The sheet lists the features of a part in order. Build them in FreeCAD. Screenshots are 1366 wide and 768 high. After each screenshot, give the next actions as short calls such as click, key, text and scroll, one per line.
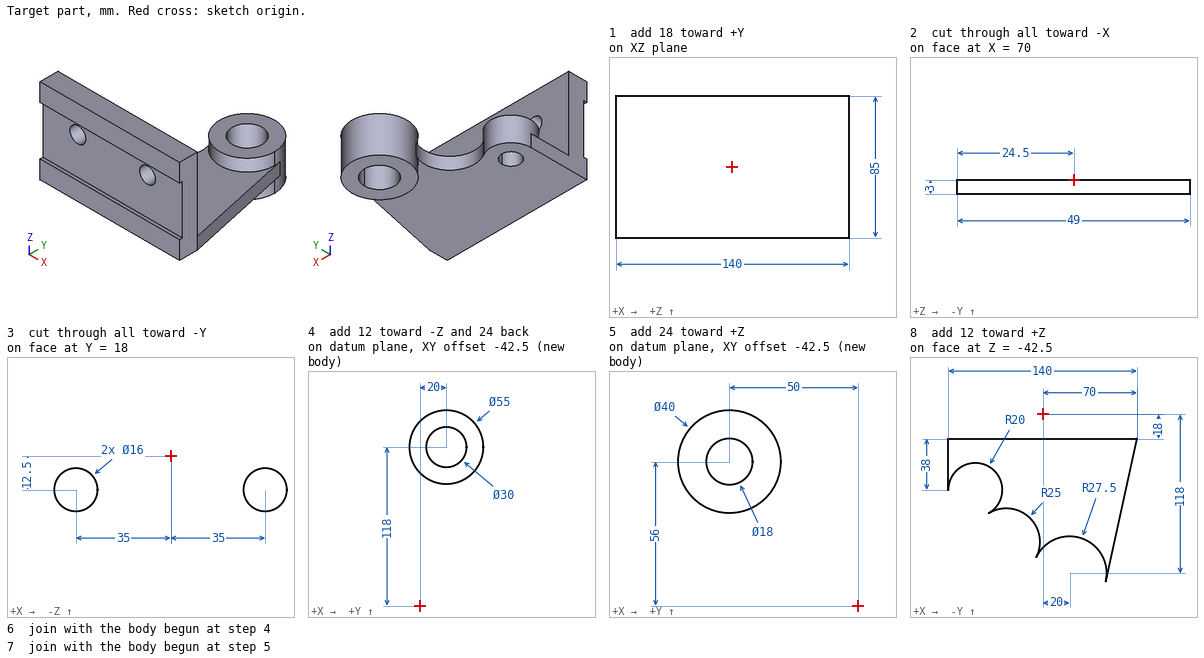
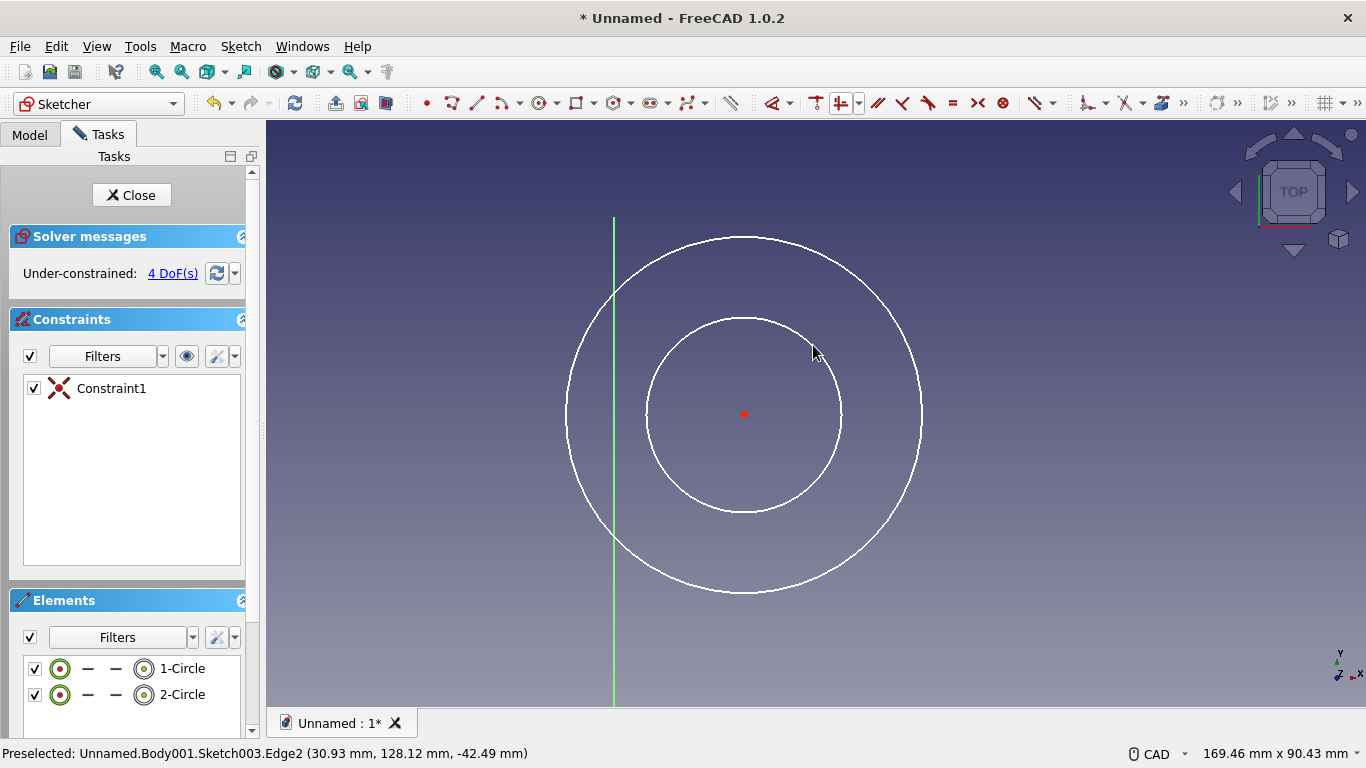
click(772, 104)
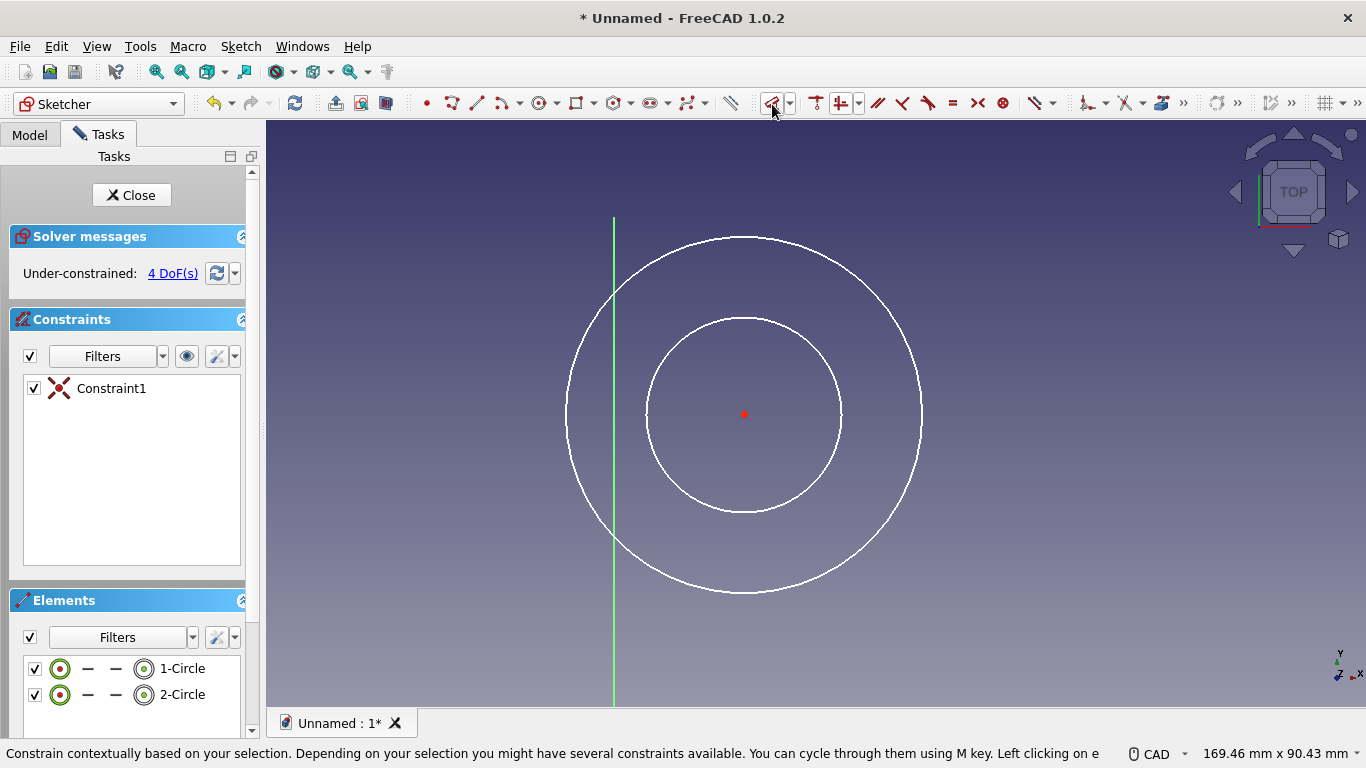
click(870, 289)
click(893, 266)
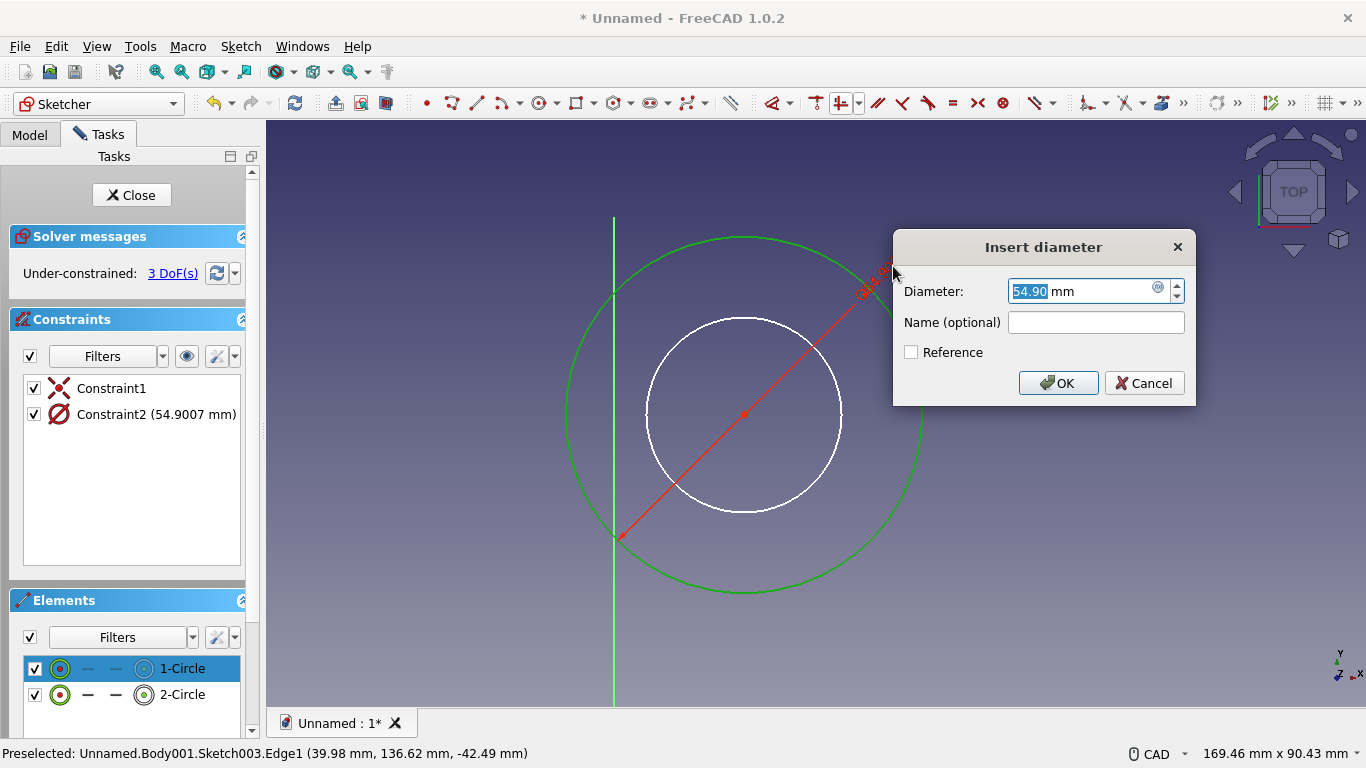
text(55)
key(Return)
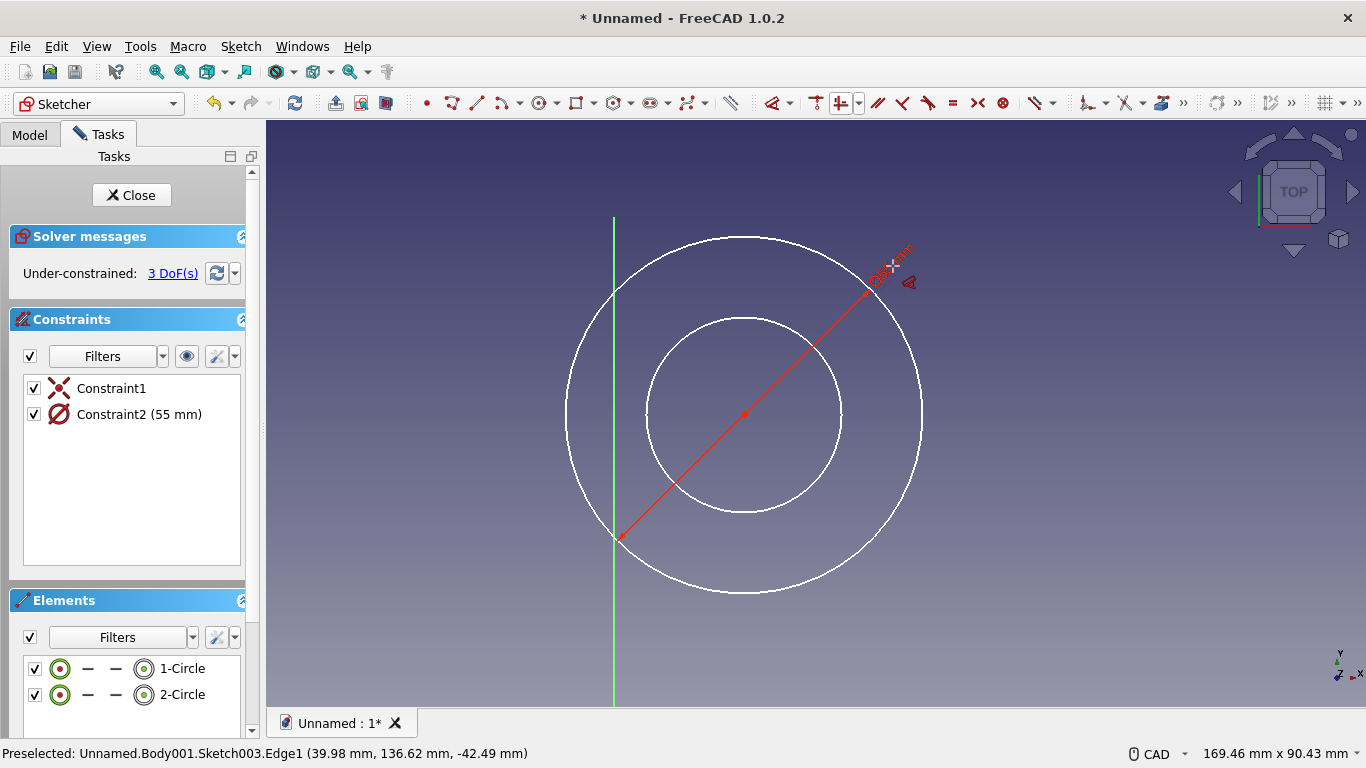
click(813, 346)
click(836, 323)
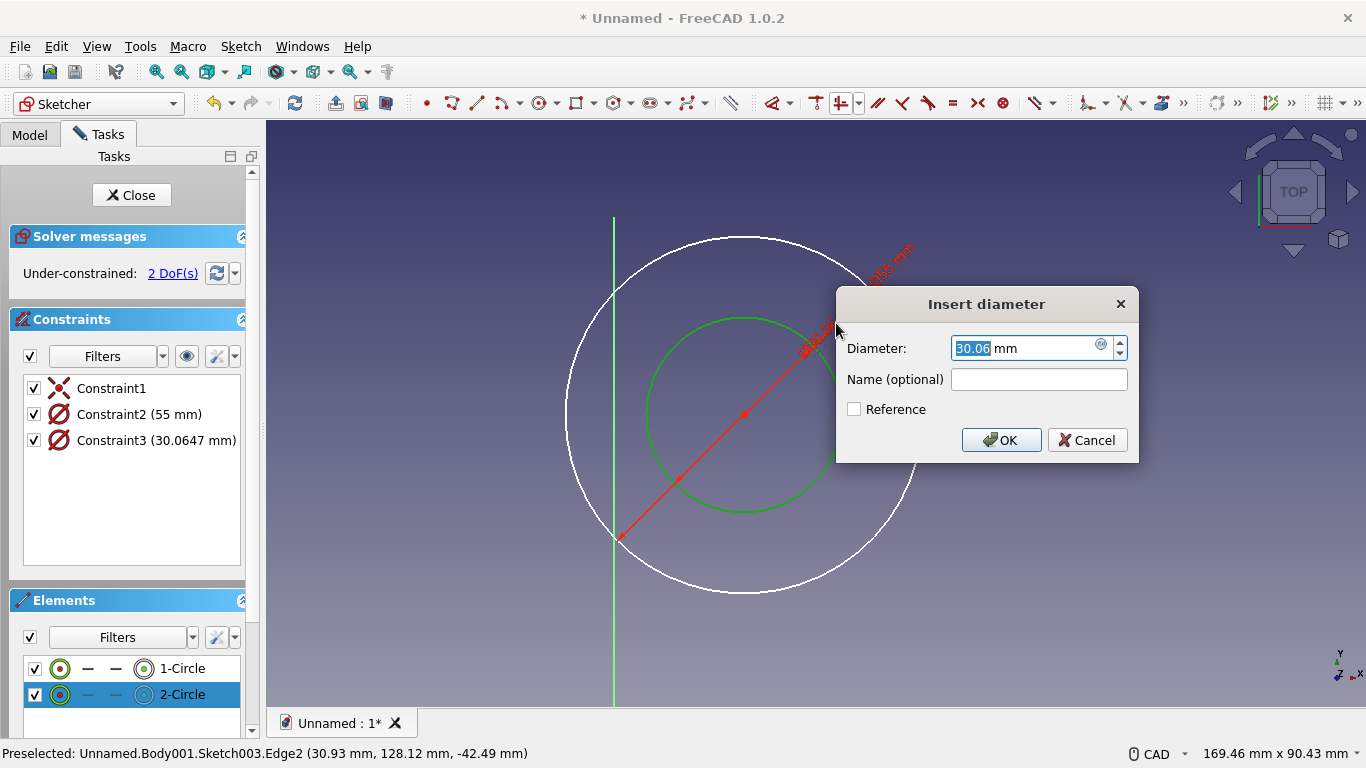
text(30)
key(Return)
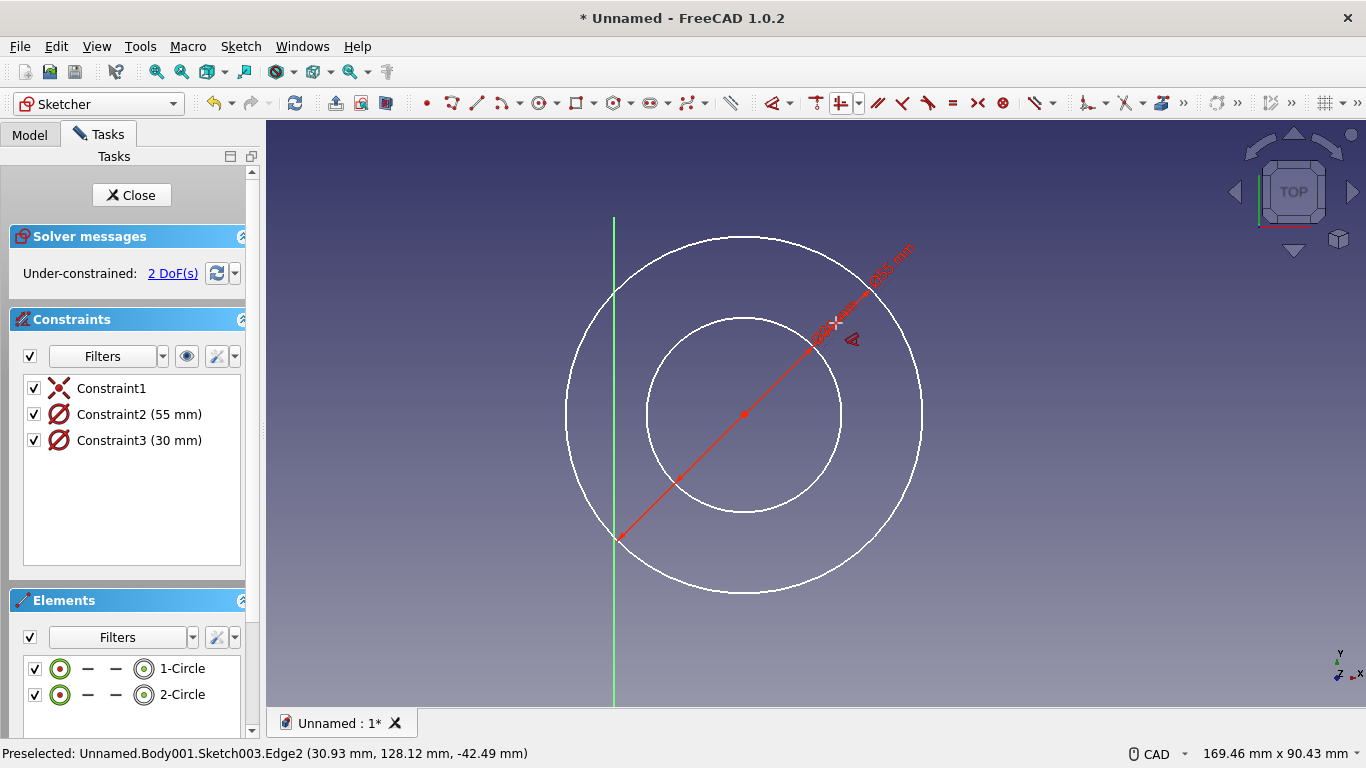
click(744, 415)
click(679, 381)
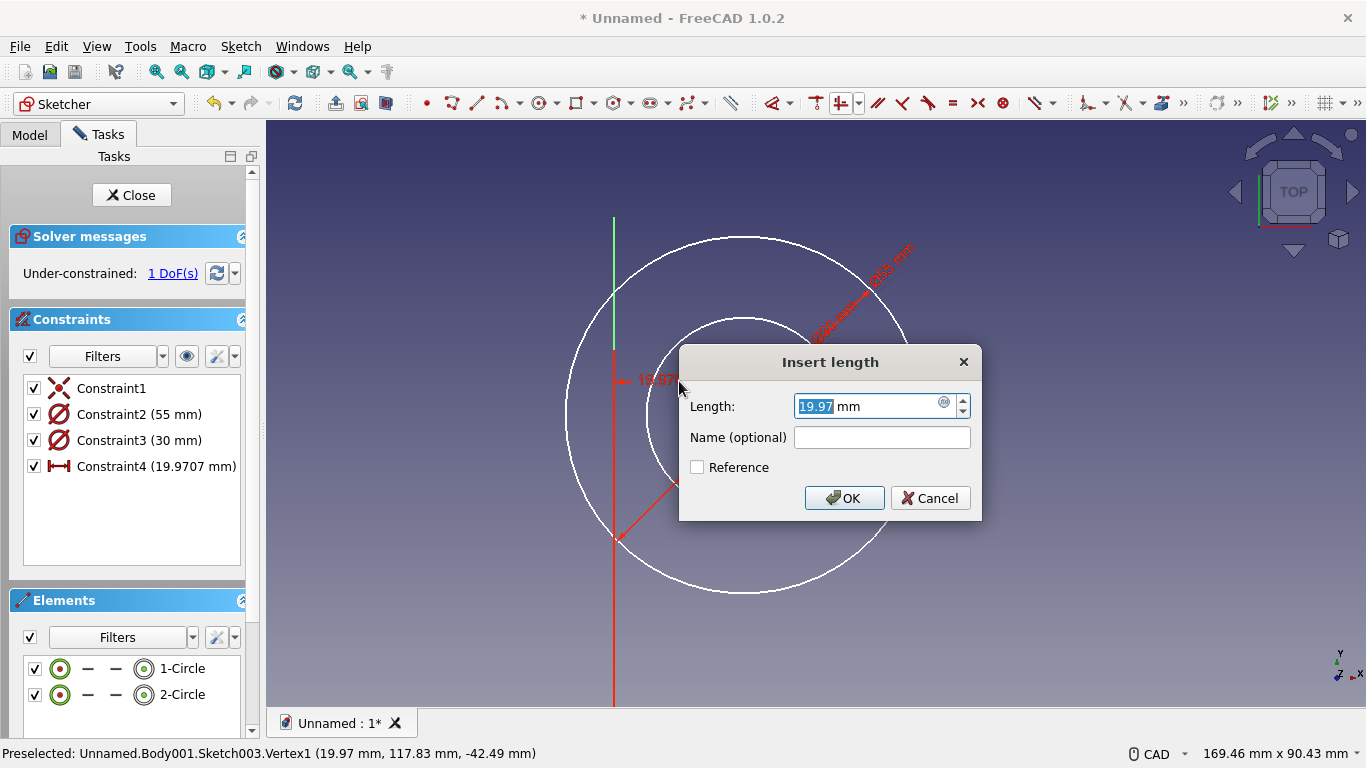
text(20)
key(Return)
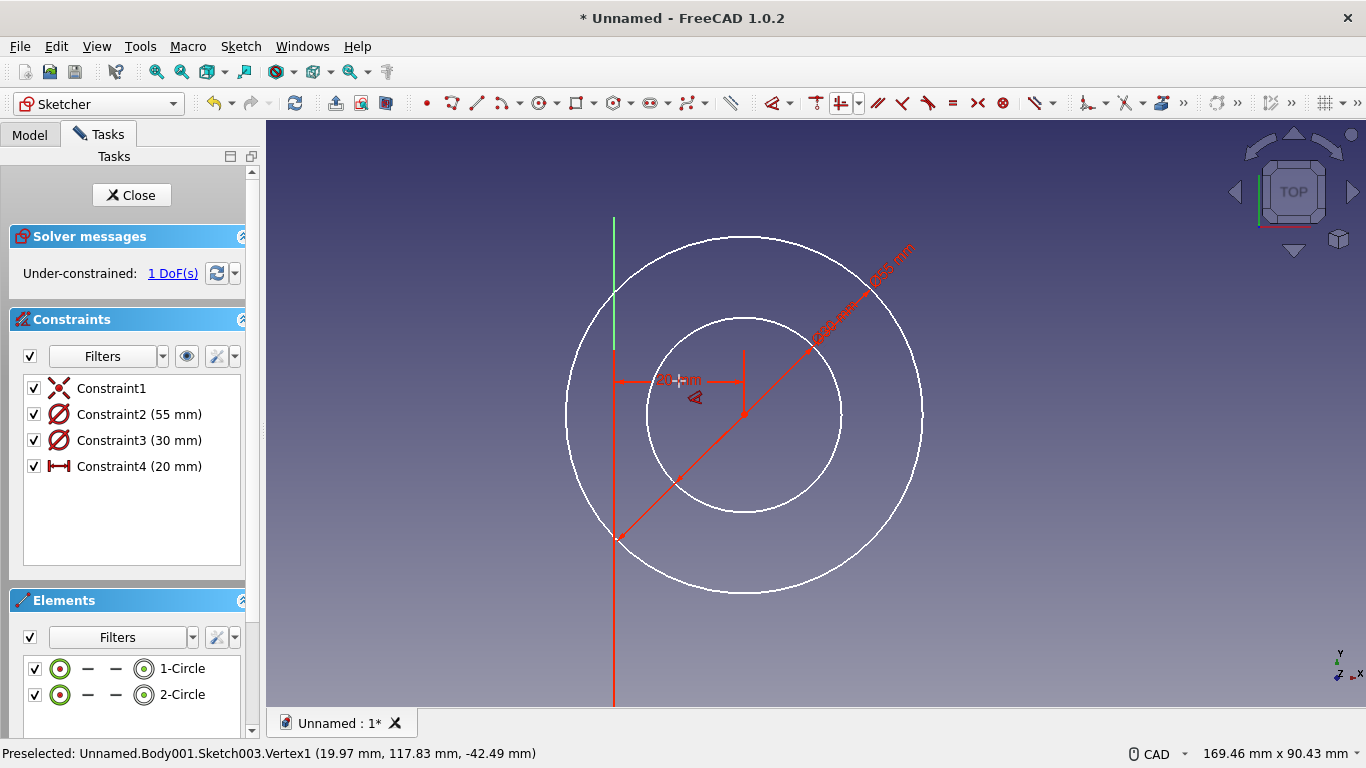
click(744, 415)
click(580, 547)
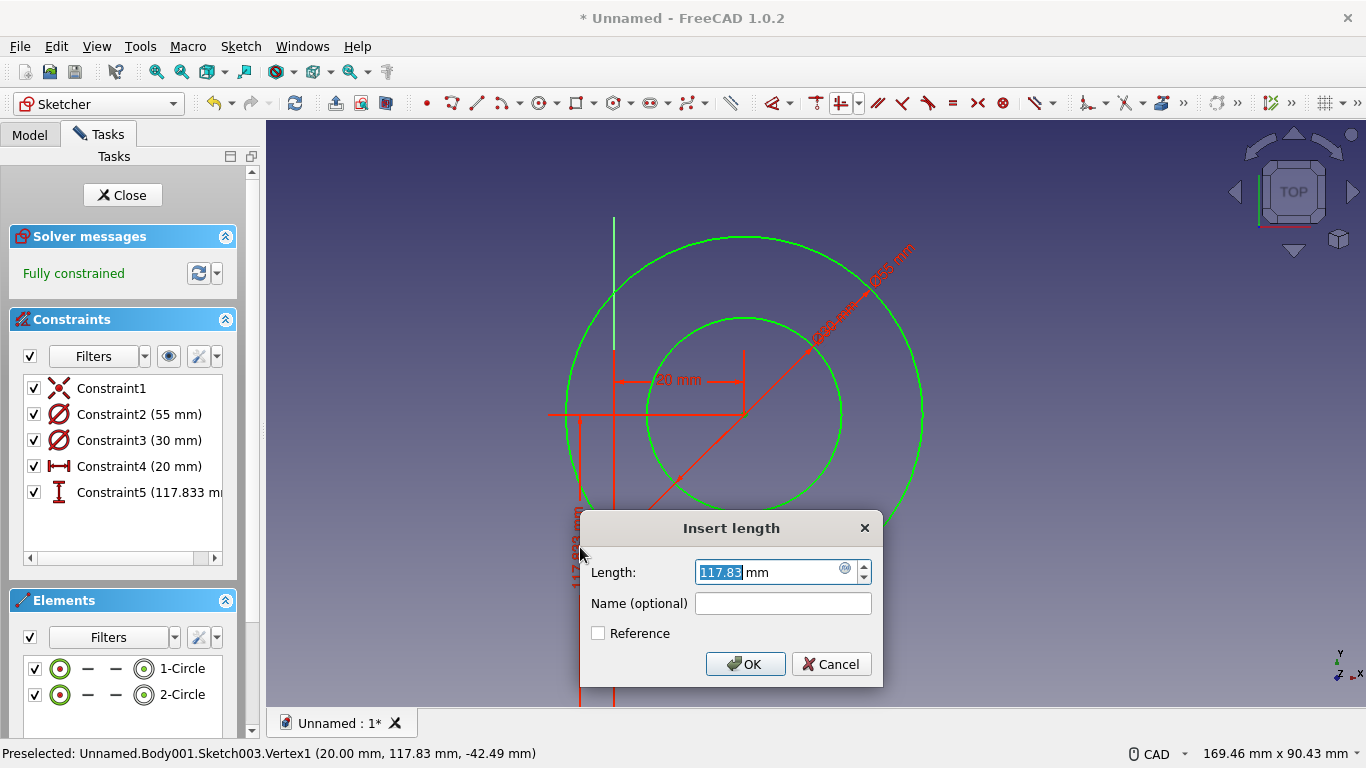
text(118)
key(Return)
key(Escape)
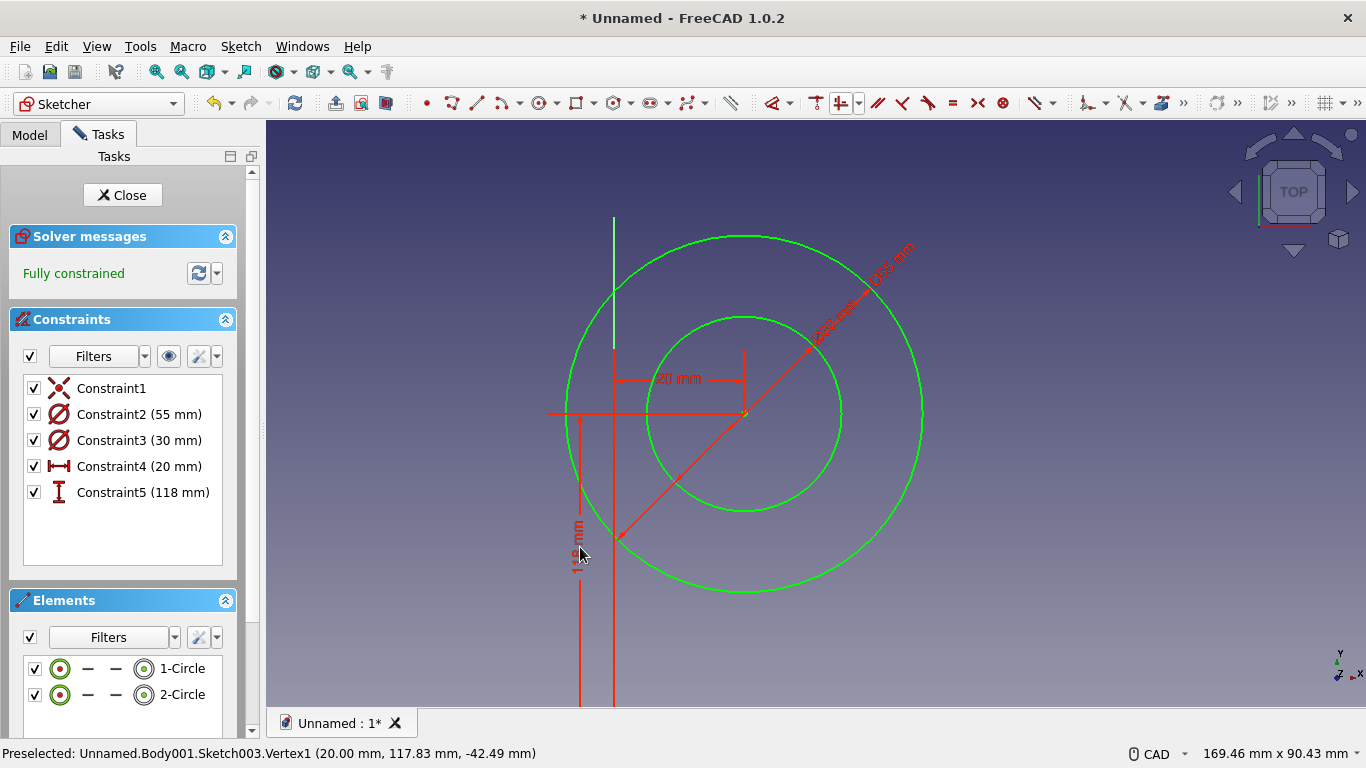
click(123, 195)